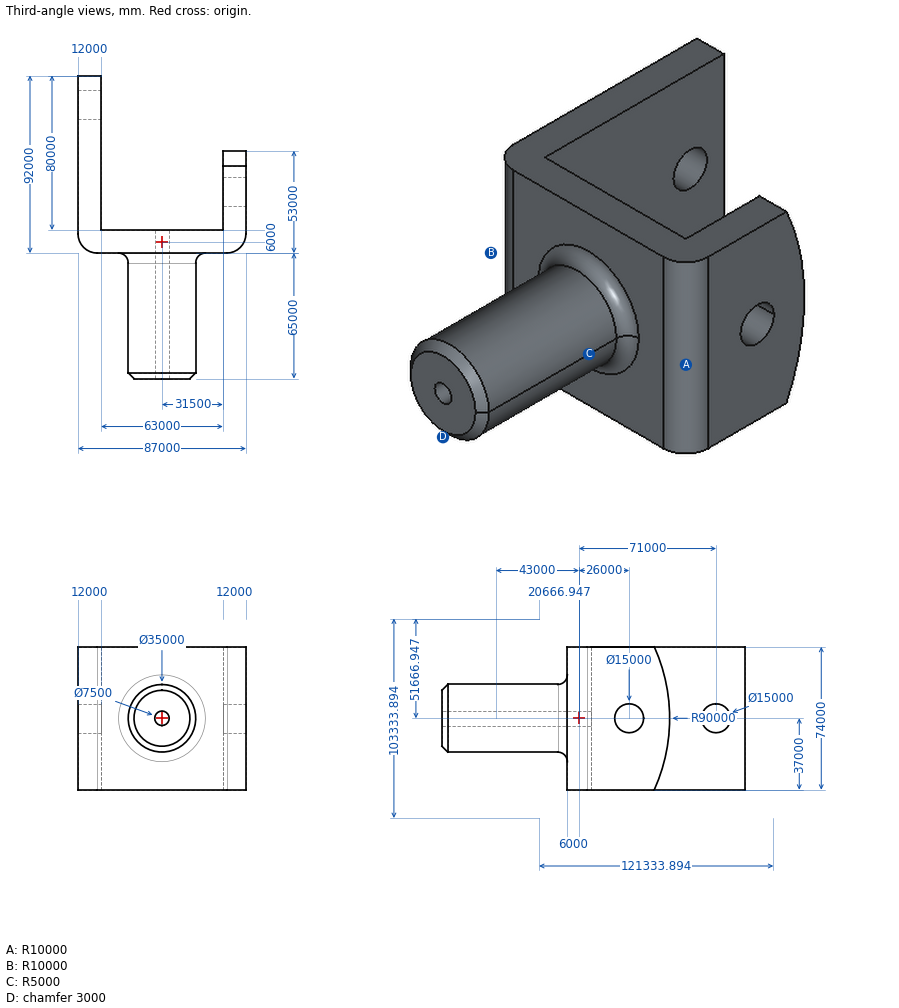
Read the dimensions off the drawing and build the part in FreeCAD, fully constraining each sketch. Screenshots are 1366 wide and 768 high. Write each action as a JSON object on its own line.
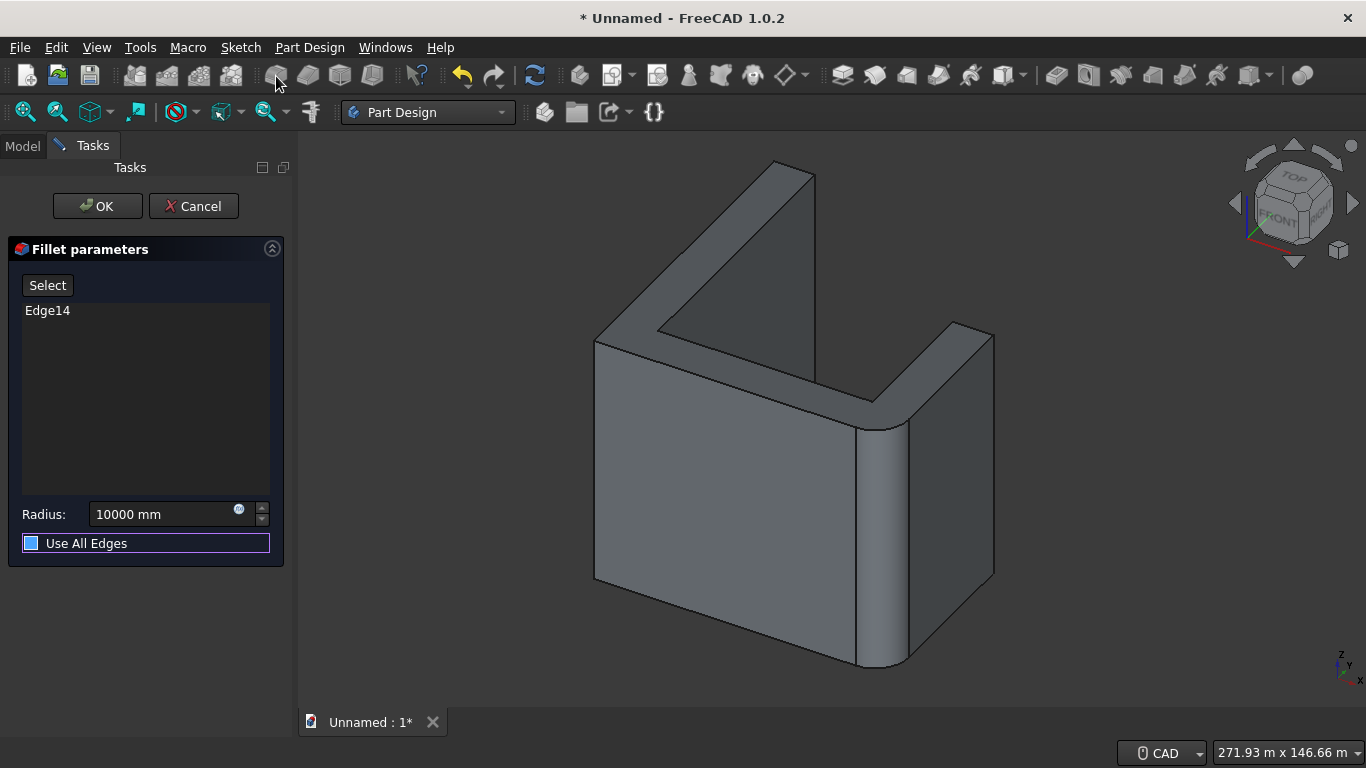
{"action": "left_click", "coordinate": [98, 206]}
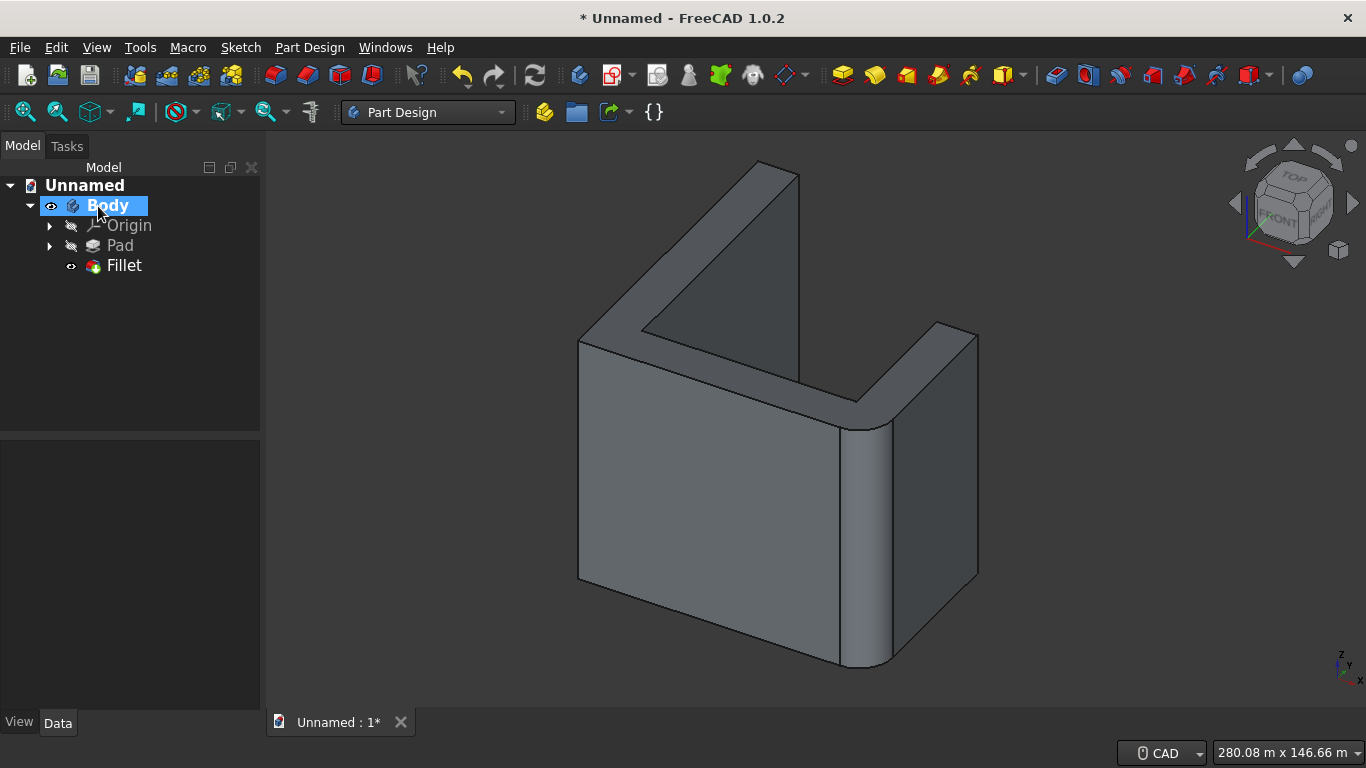
{"action": "key", "text": "0"}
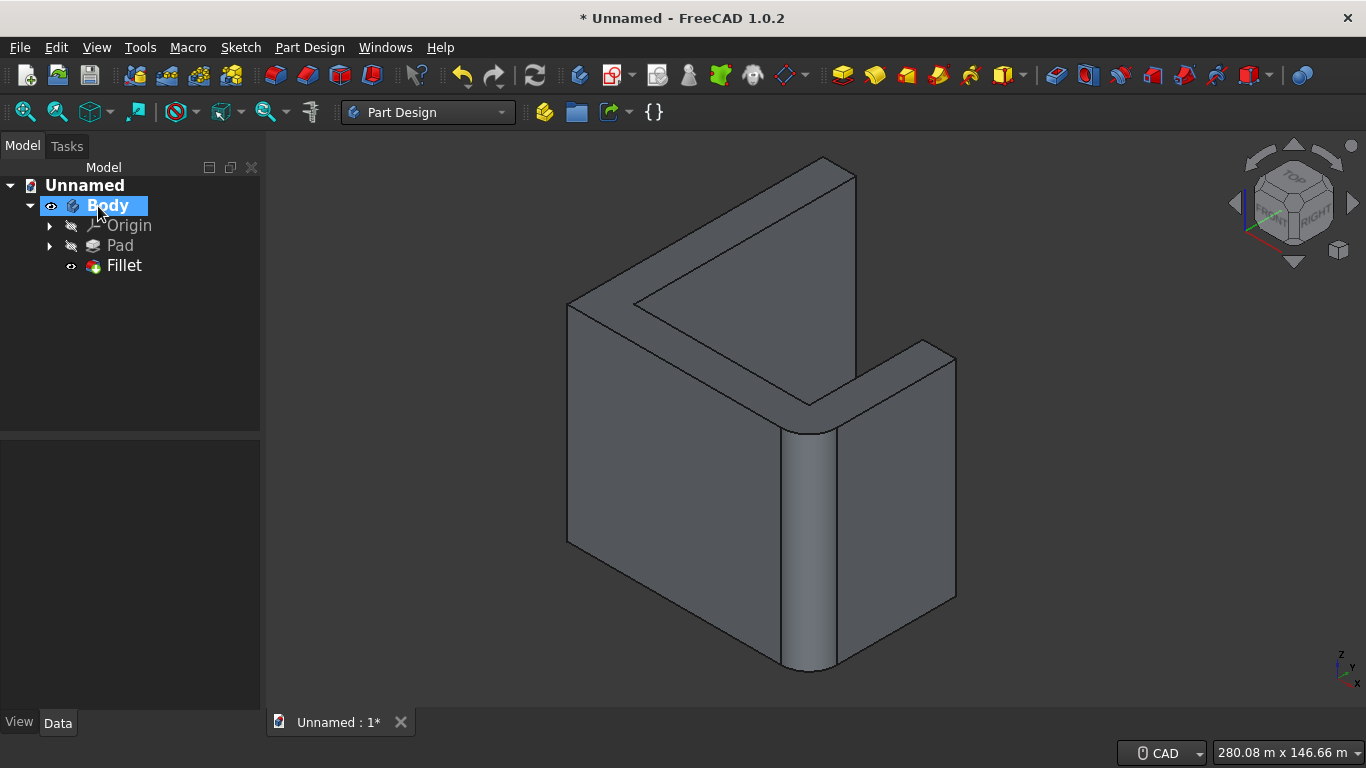
{"action": "key", "text": "2"}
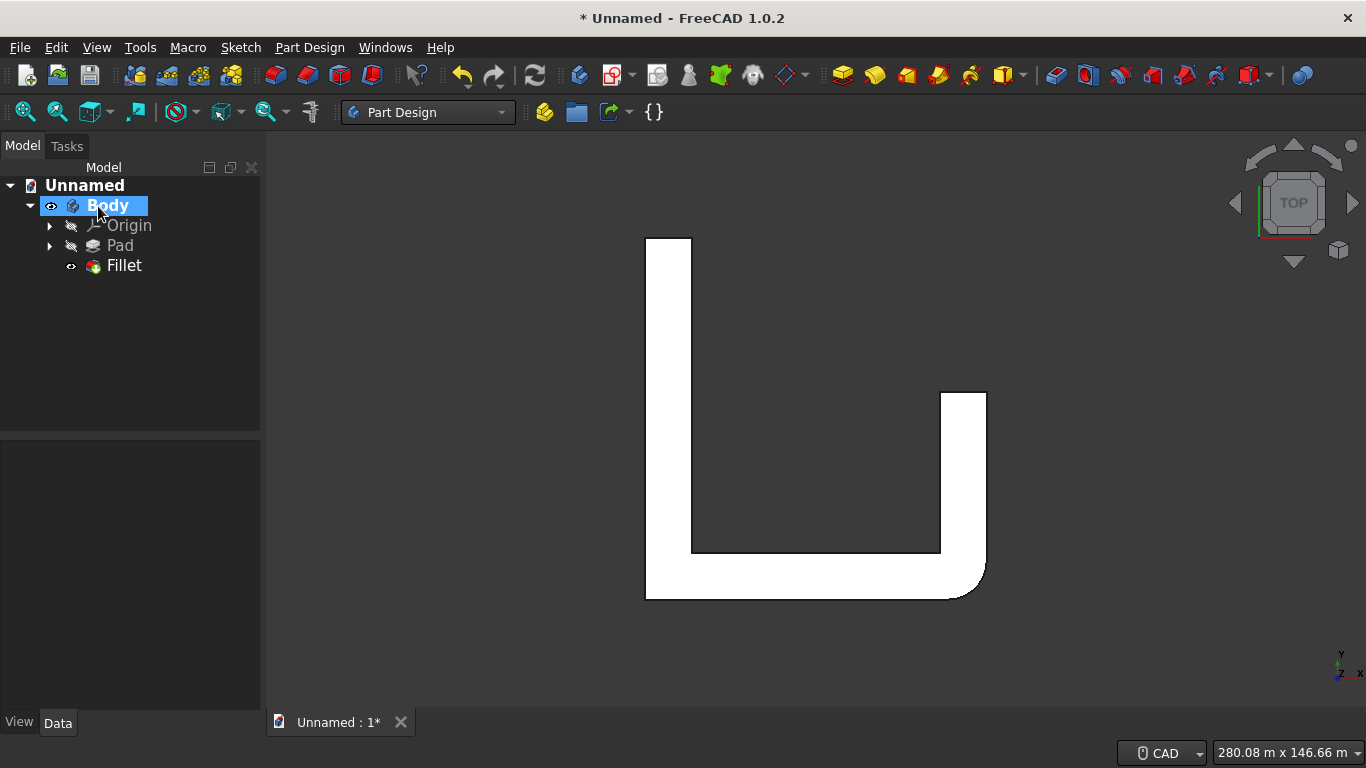
{"action": "key", "text": "1"}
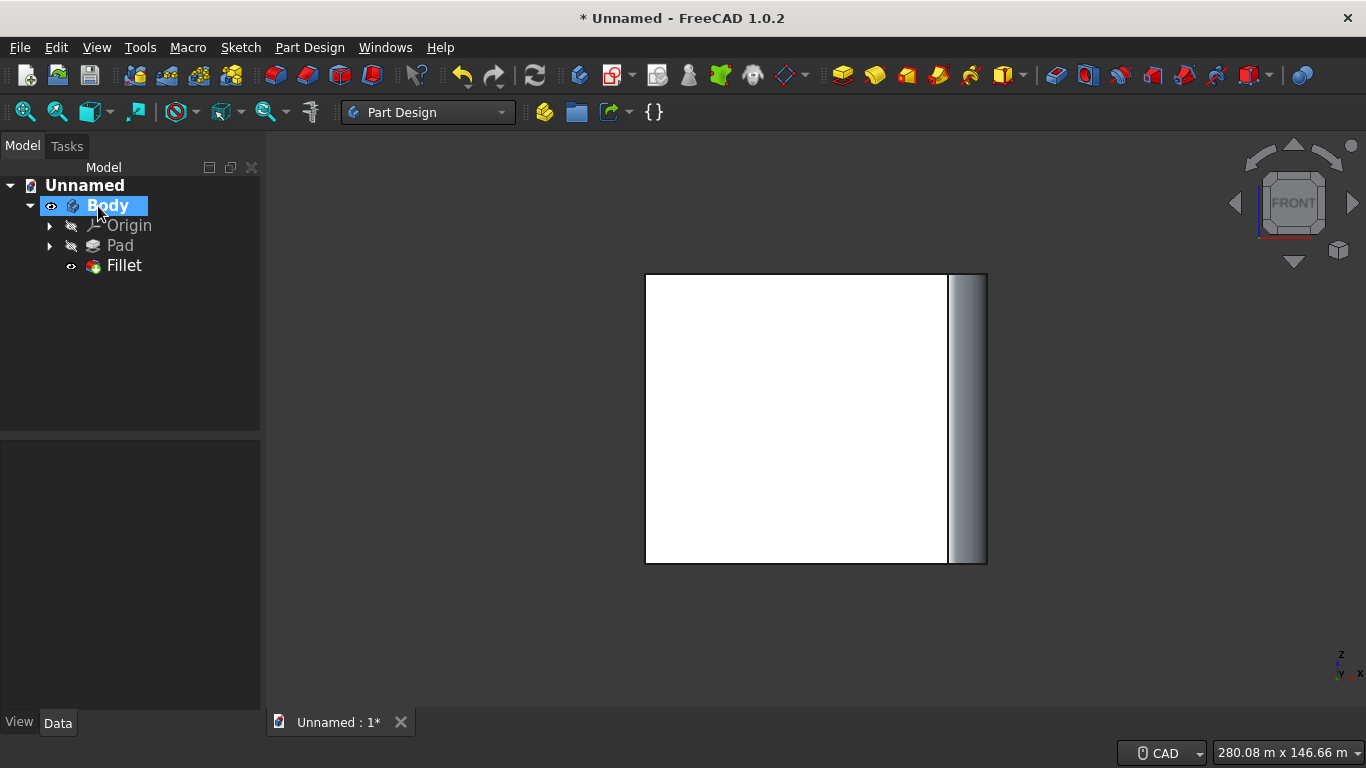
{"action": "left_click", "coordinate": [645, 418]}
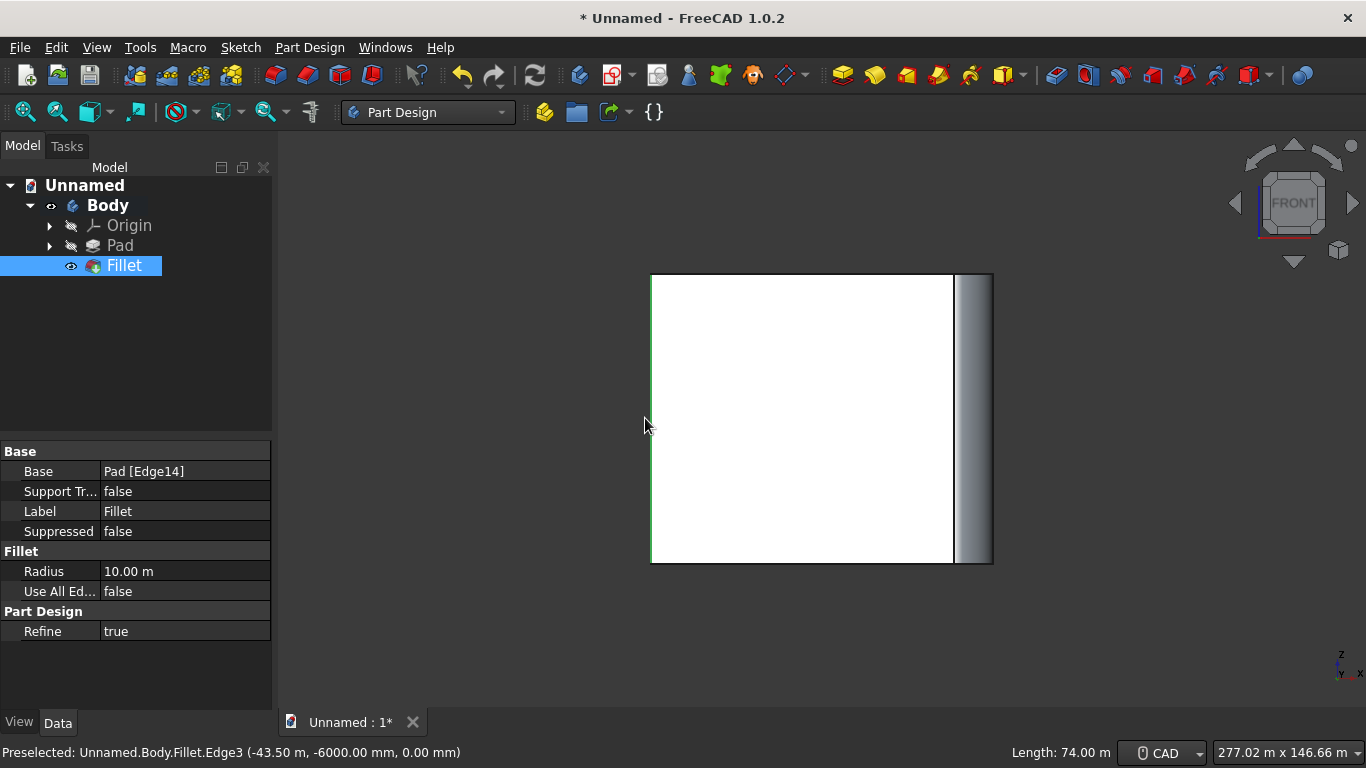
{"action": "left_click", "coordinate": [276, 76]}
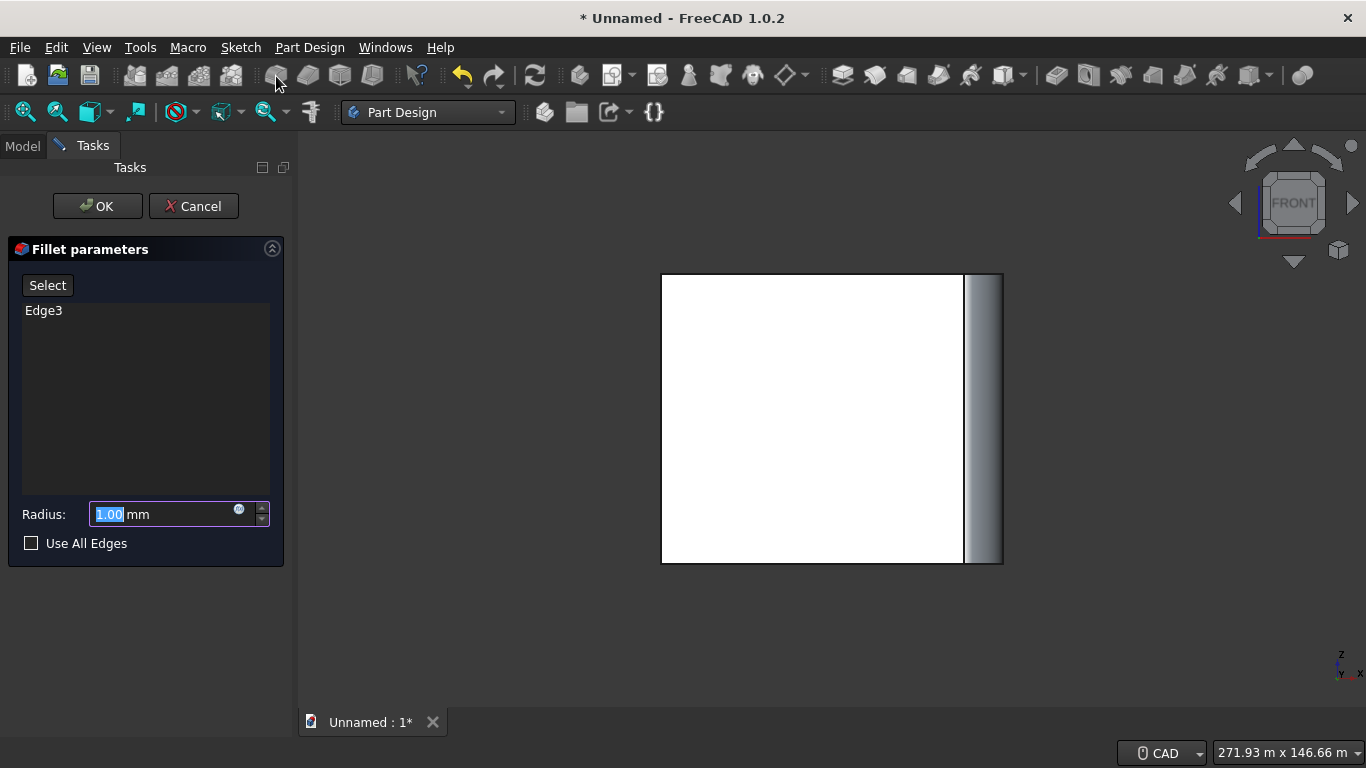
{"action": "type", "text": "10000"}
{"action": "key", "text": "Tab"}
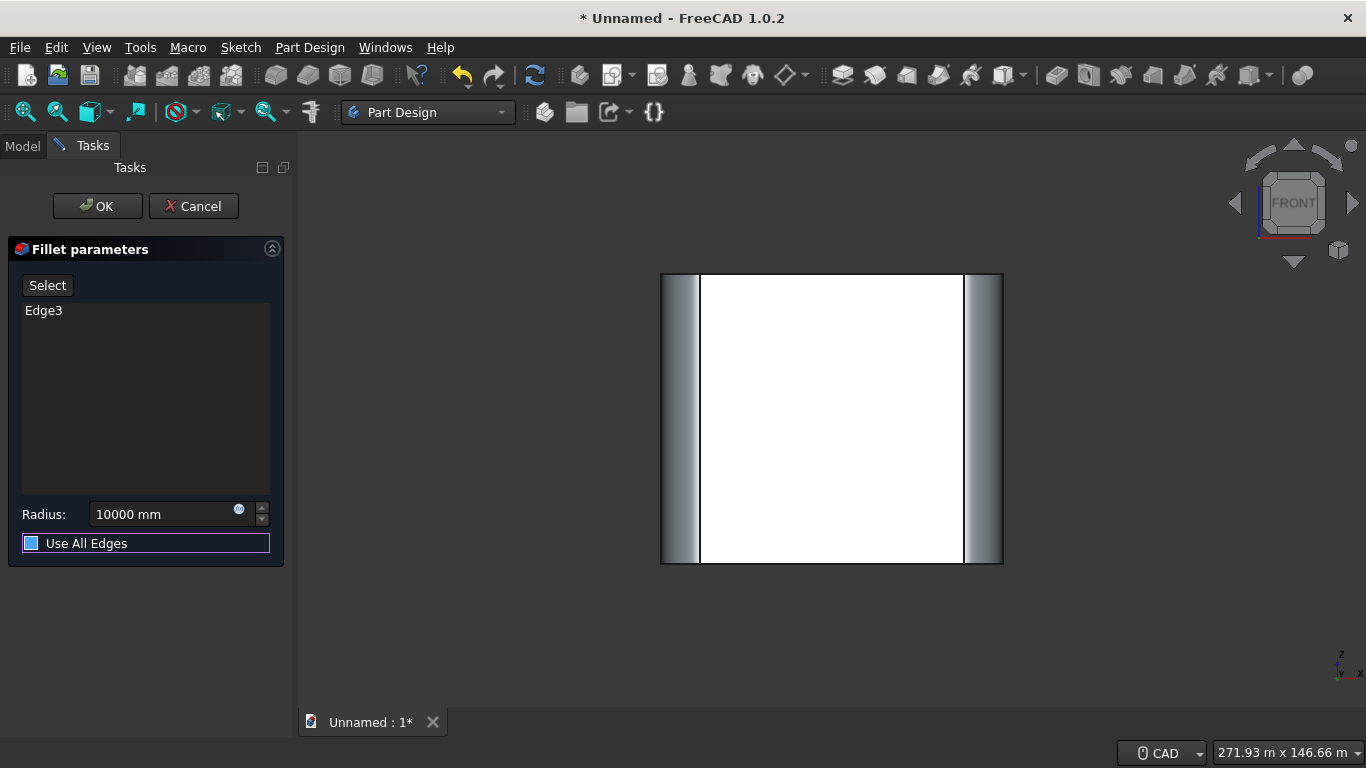
{"action": "left_click", "coordinate": [98, 206]}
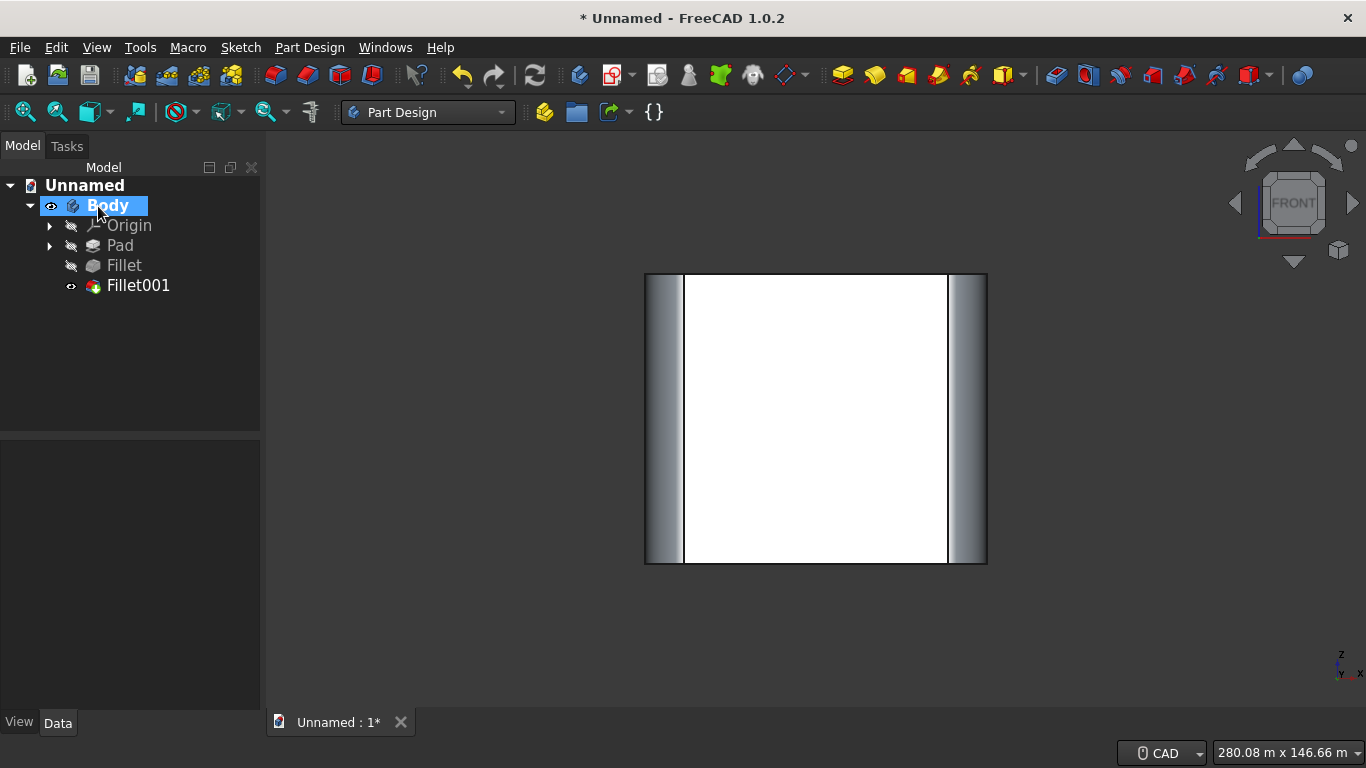
{"action": "key", "text": "0"}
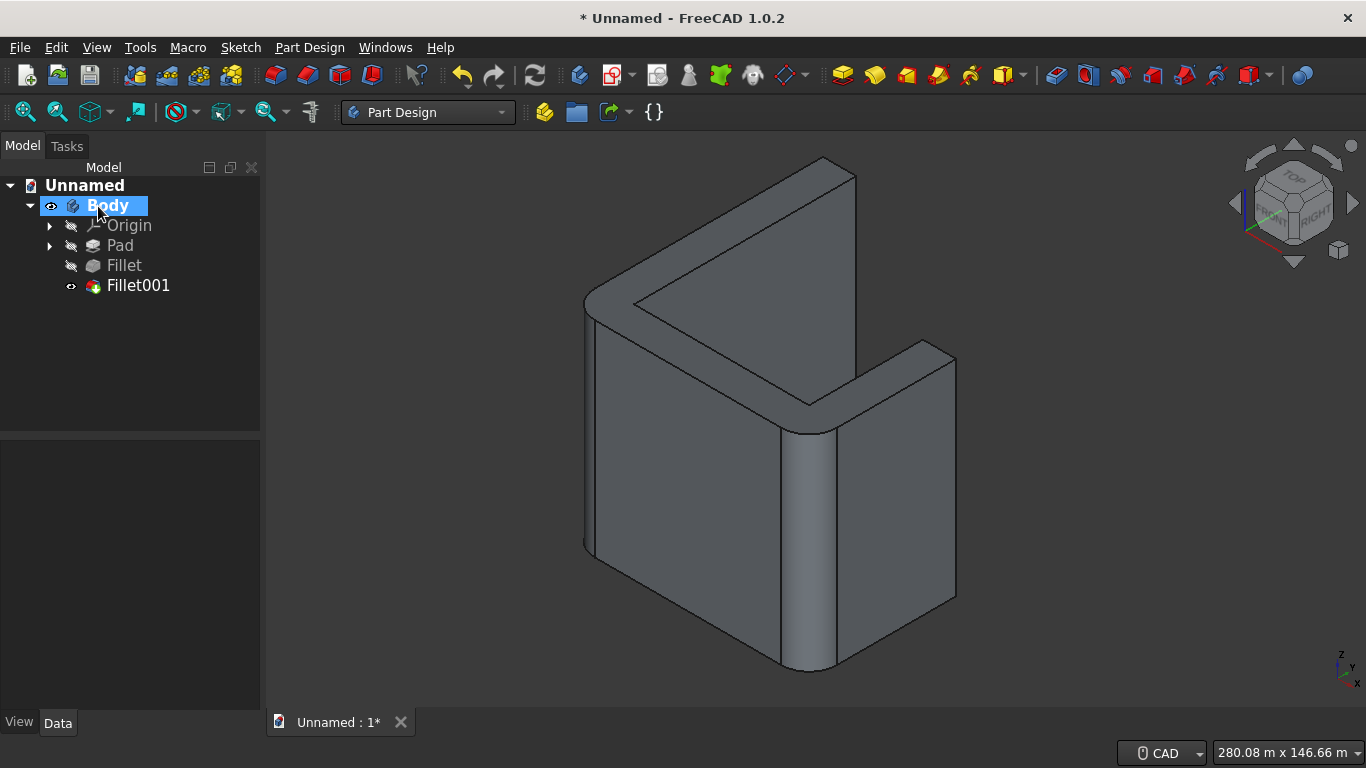
{"action": "left_click", "coordinate": [897, 477]}